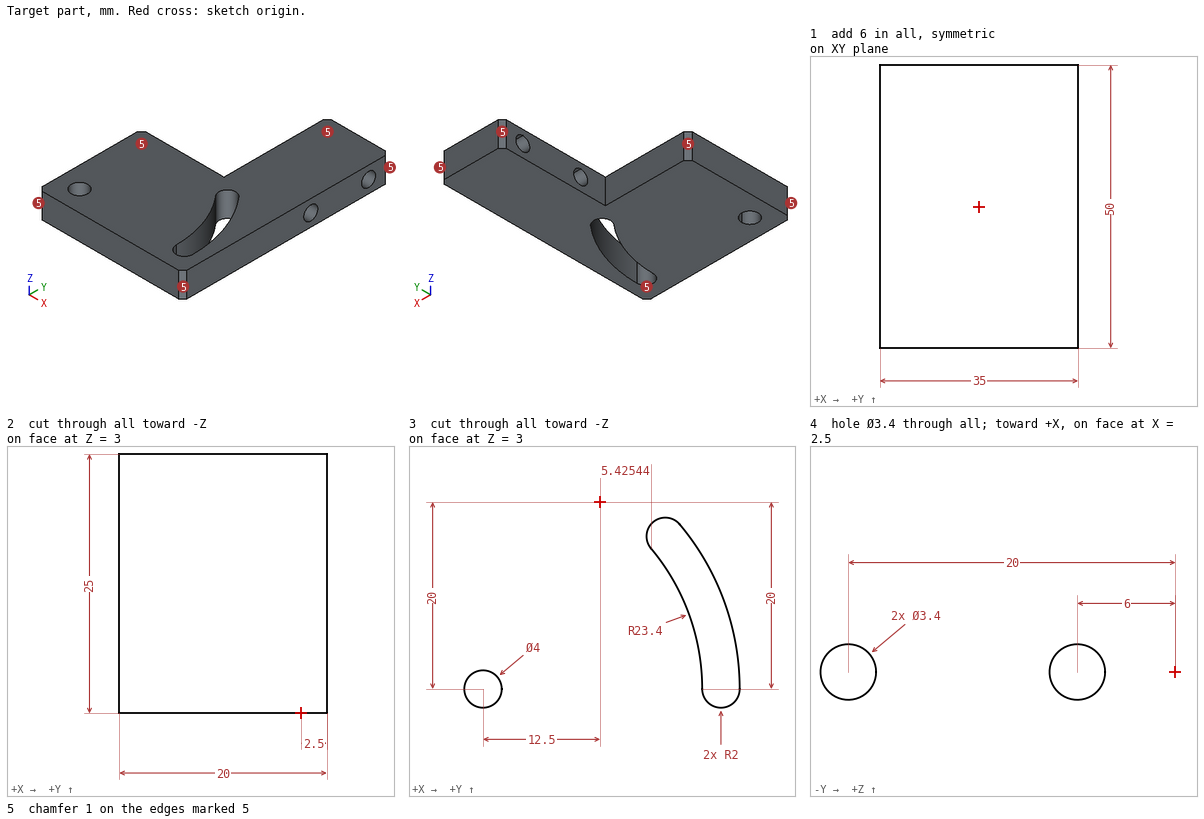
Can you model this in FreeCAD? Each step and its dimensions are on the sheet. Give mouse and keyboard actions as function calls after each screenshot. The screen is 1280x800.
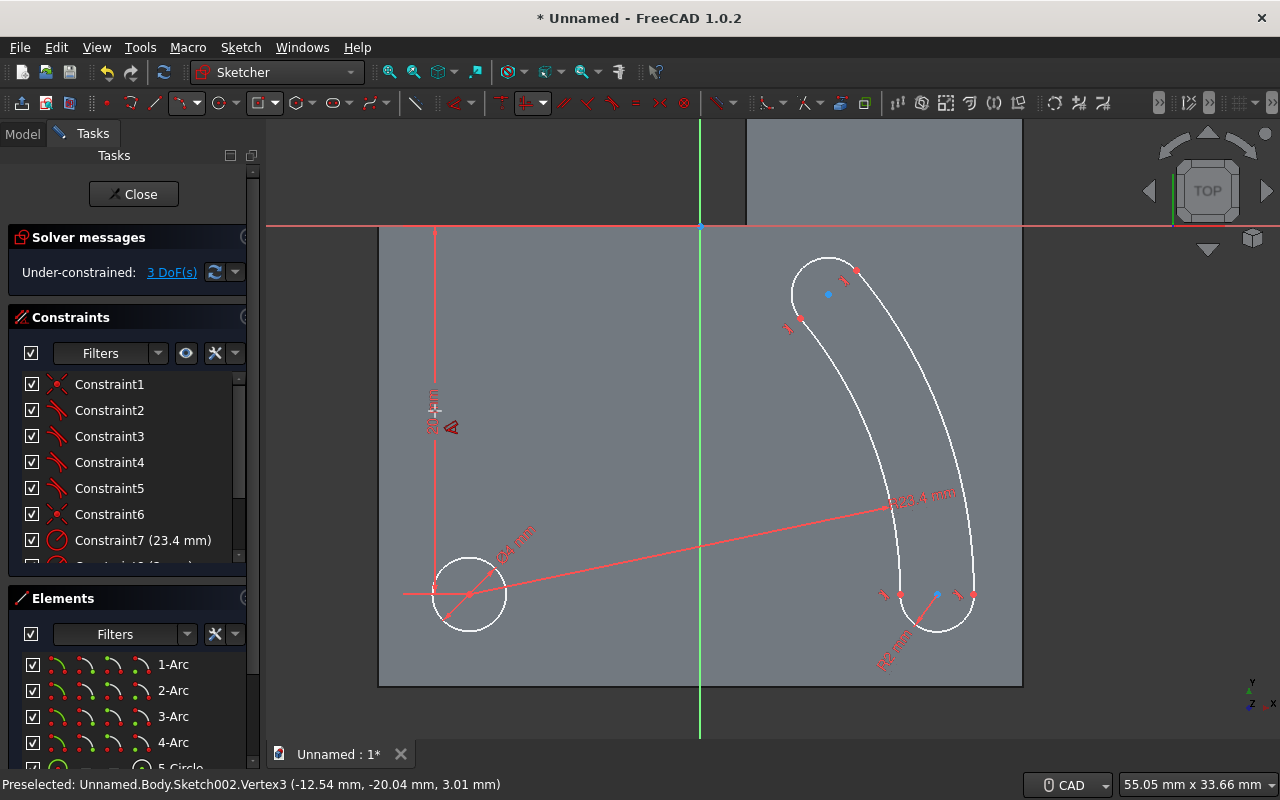
click(900, 595)
click(934, 326)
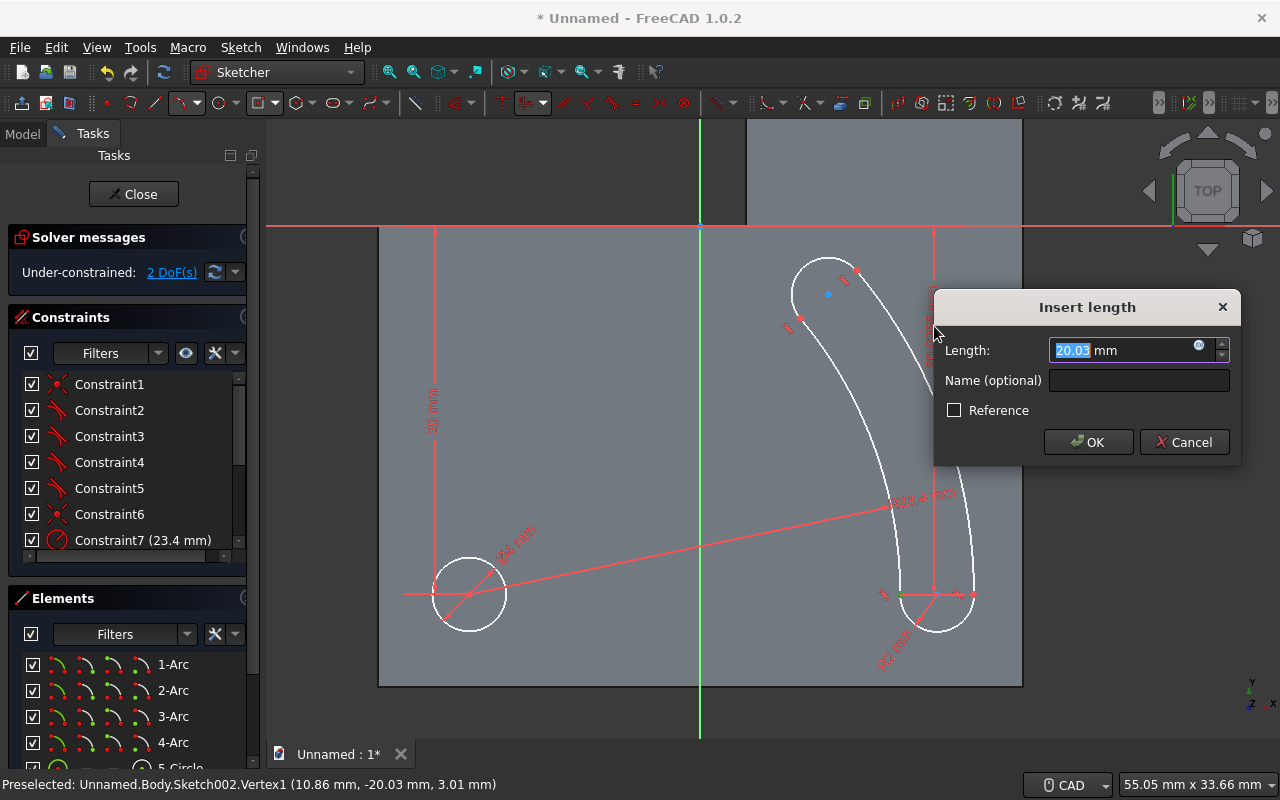
text(20)
key(Return)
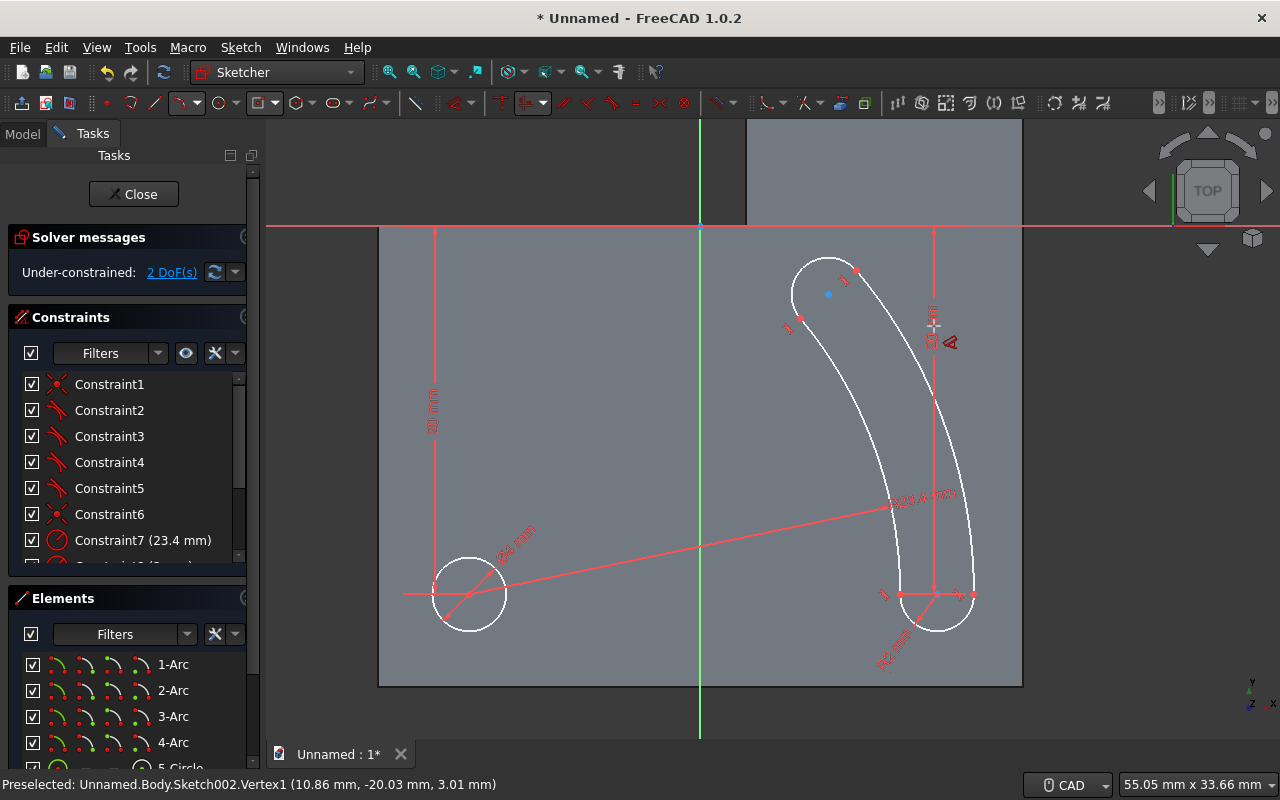
click(469, 594)
click(585, 192)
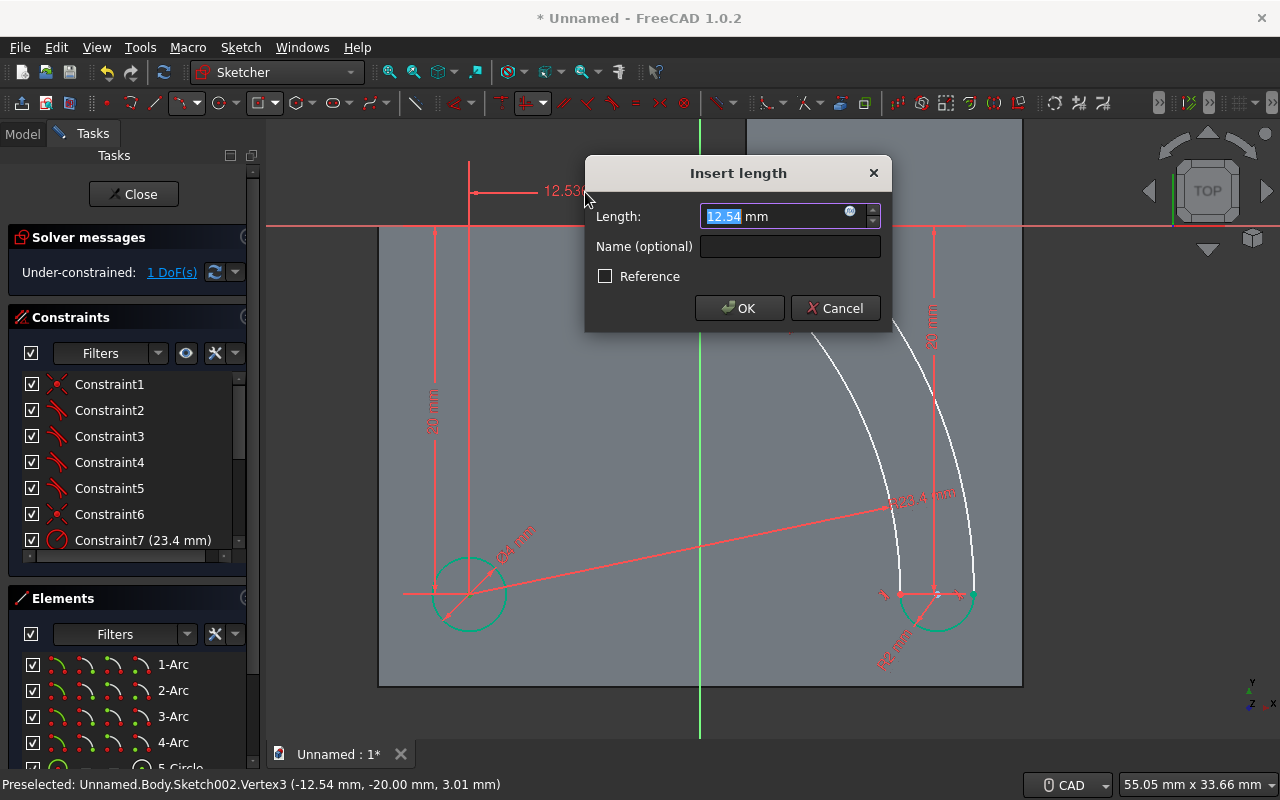
text(12.5)
key(Return)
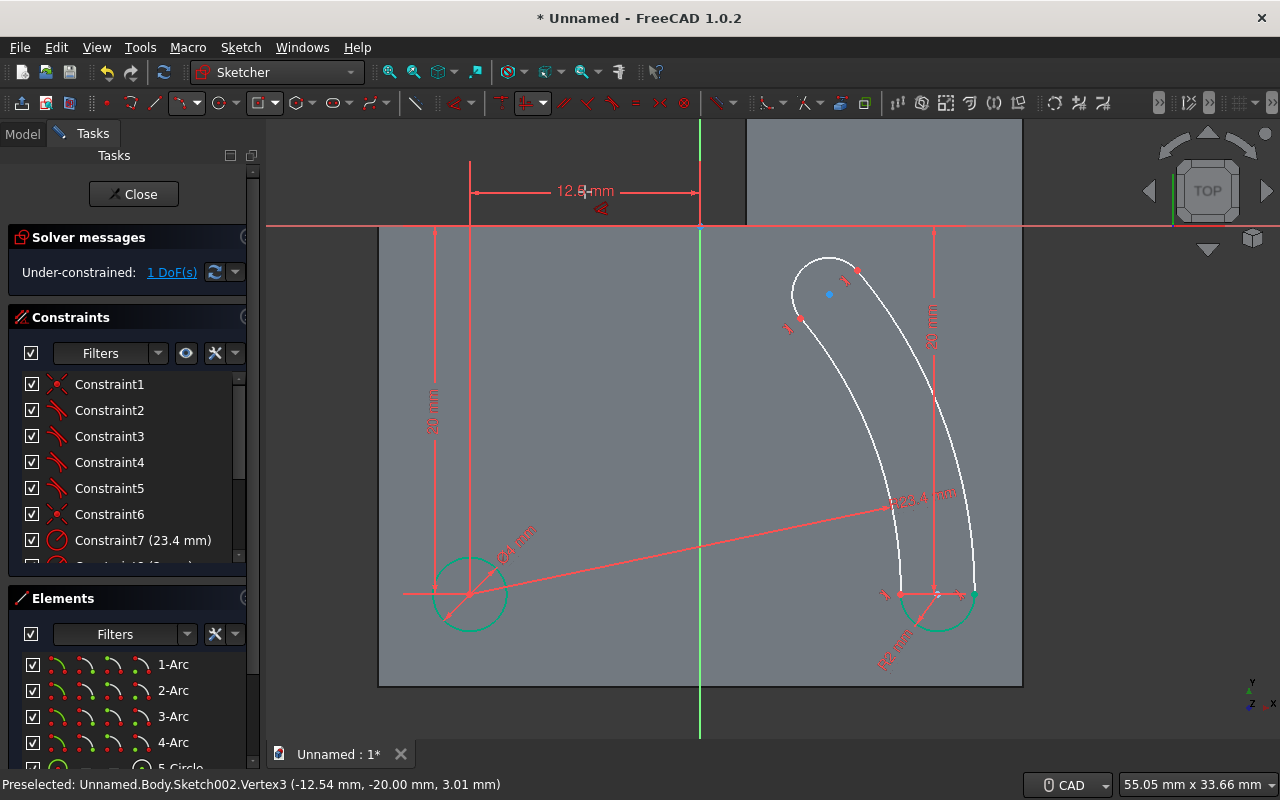
click(801, 318)
click(750, 192)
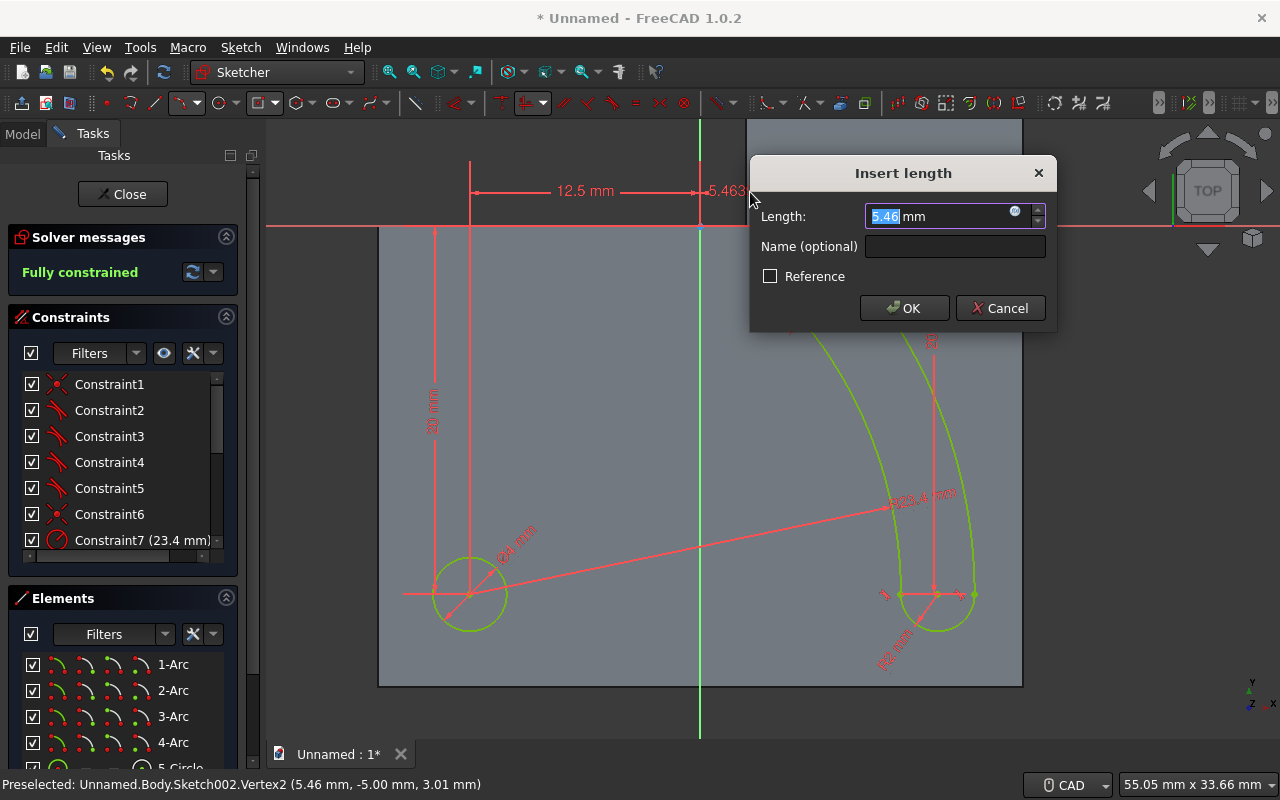
text(5.42544)
key(Return)
key(Escape)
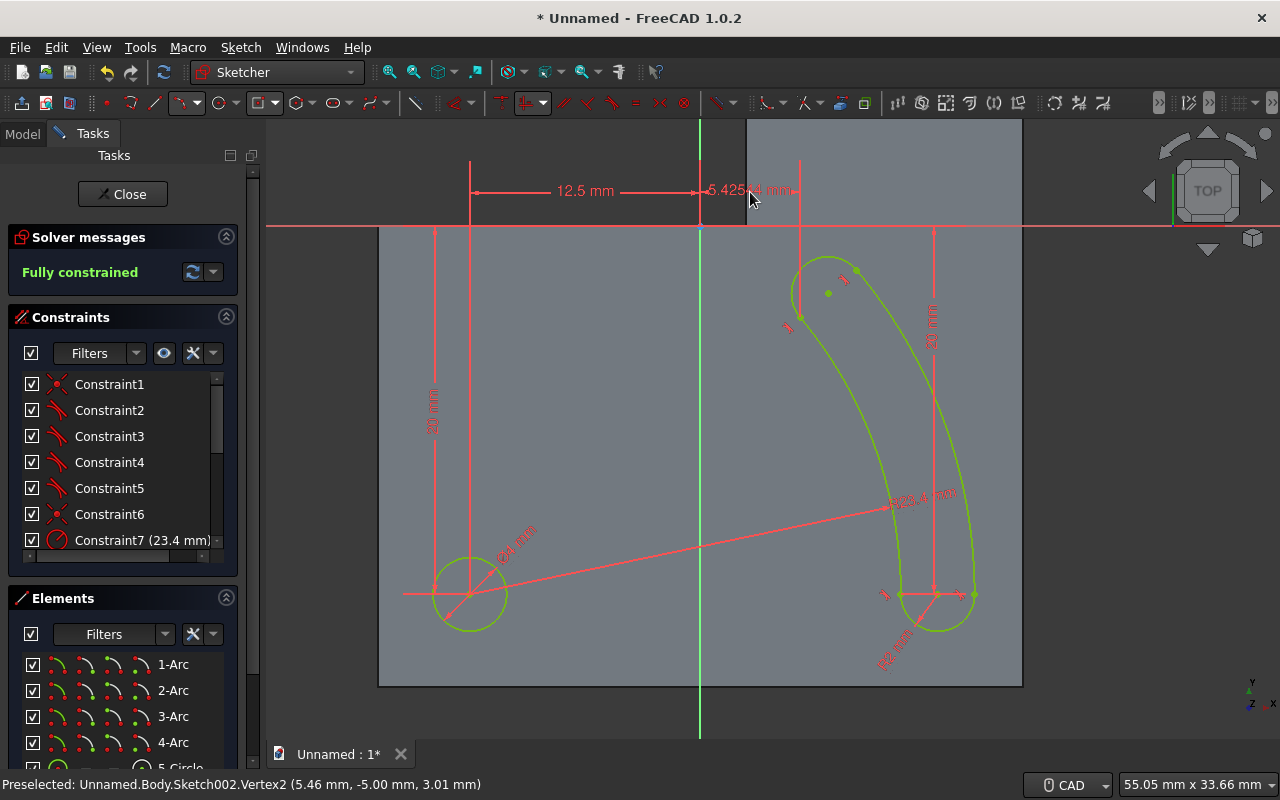
click(123, 194)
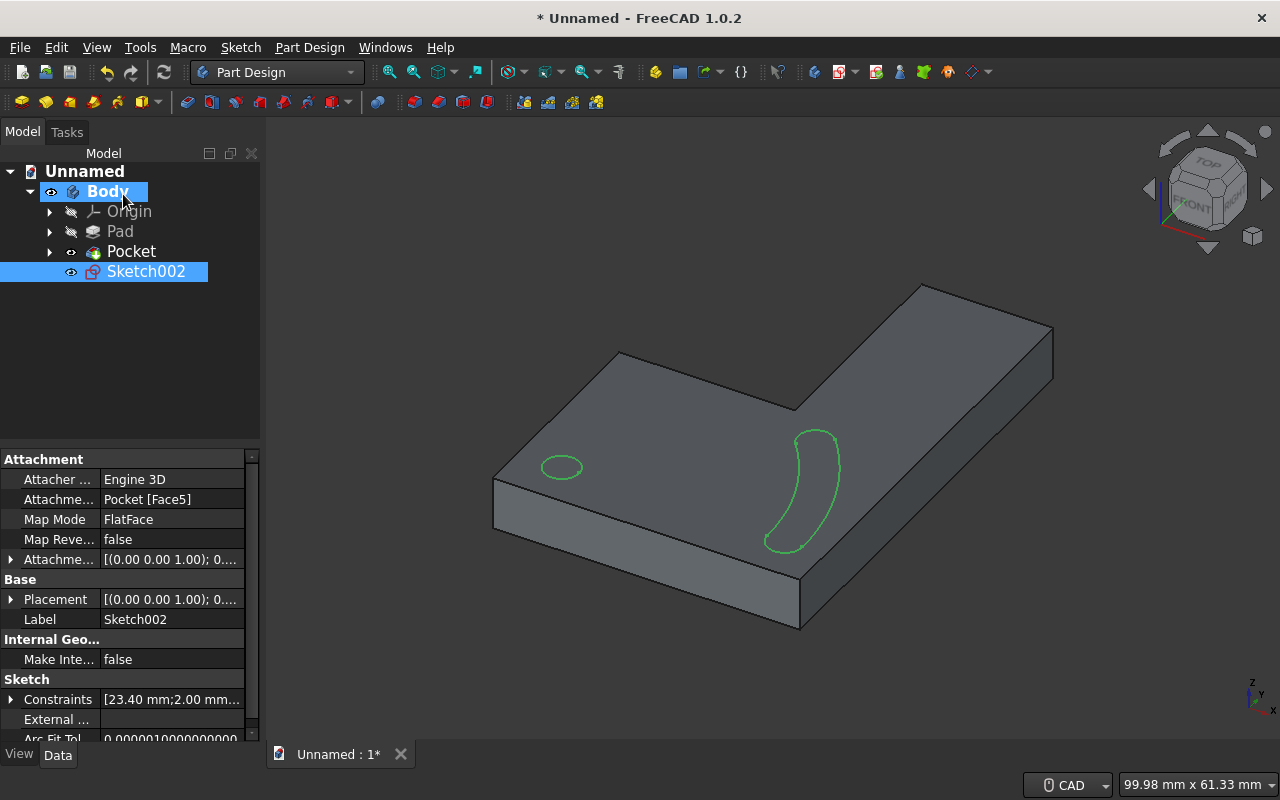
click(188, 102)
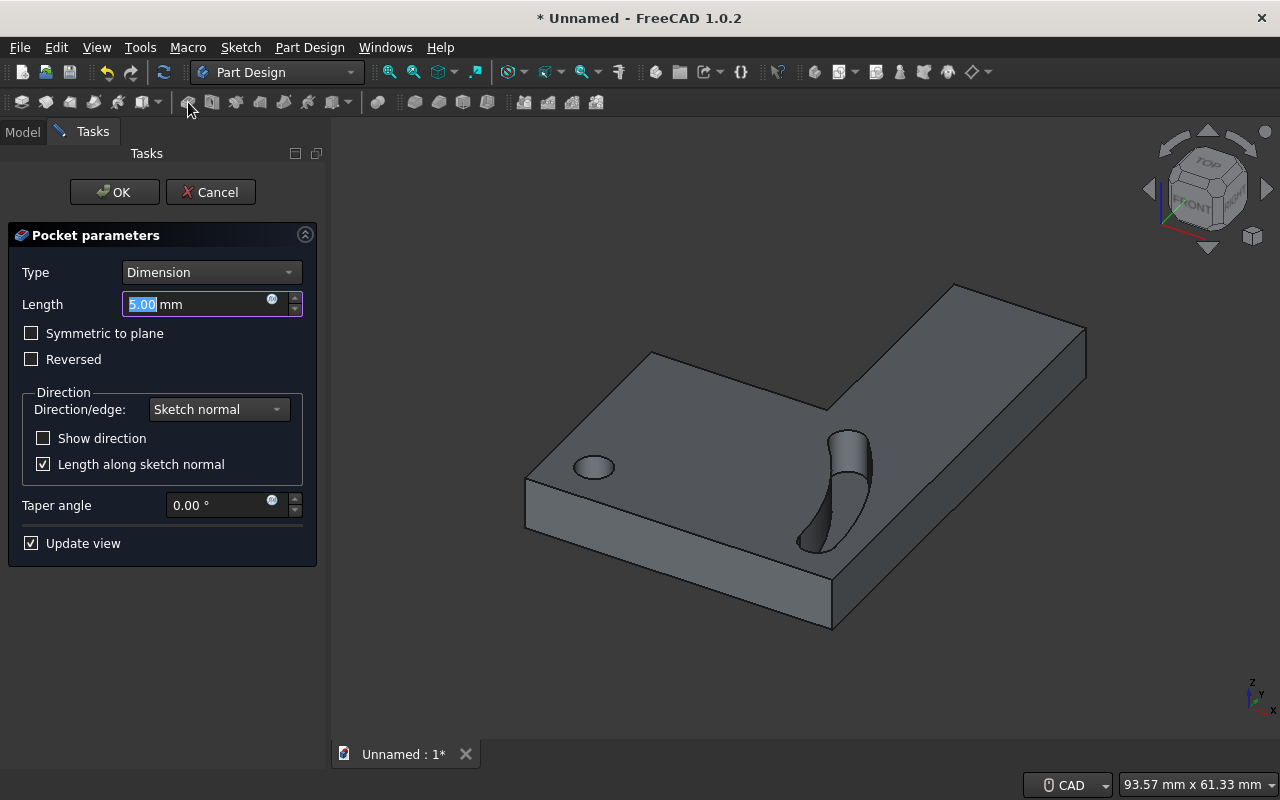
click(212, 272)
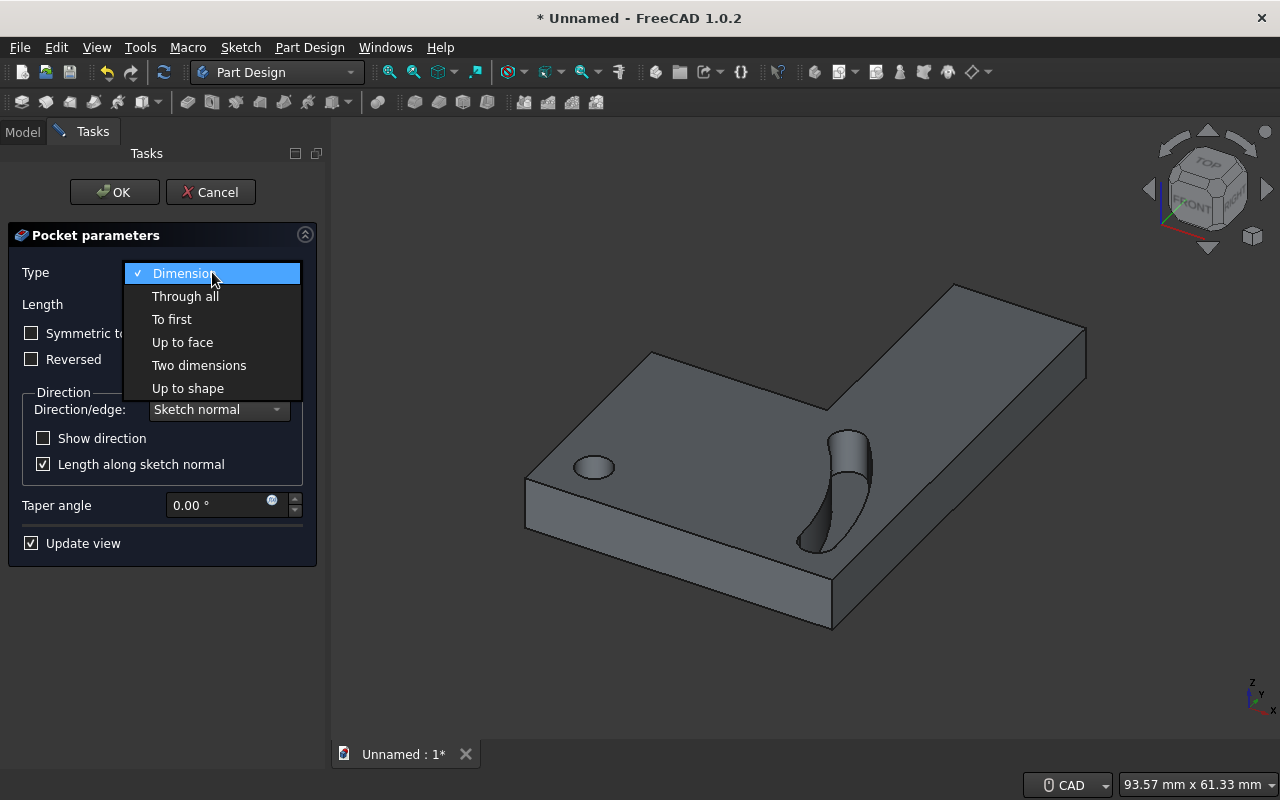
click(212, 296)